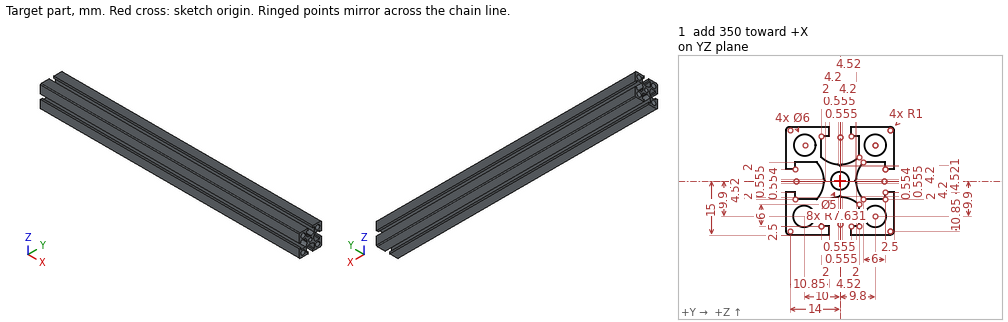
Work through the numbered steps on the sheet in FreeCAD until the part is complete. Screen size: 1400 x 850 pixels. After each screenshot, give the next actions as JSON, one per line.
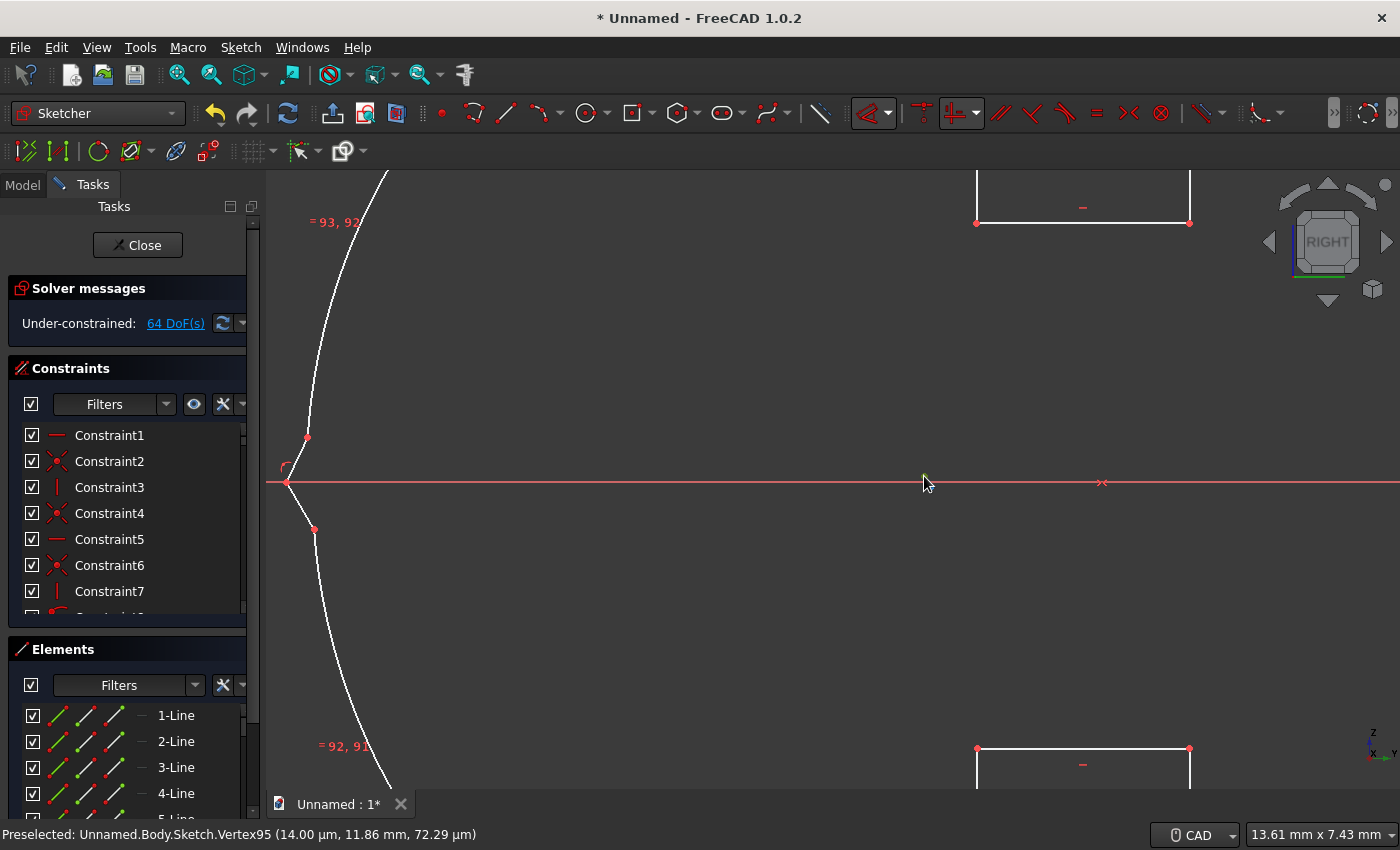
{"action": "scroll", "coordinate": [929, 479], "scroll_direction": "down", "scroll_amount": 9}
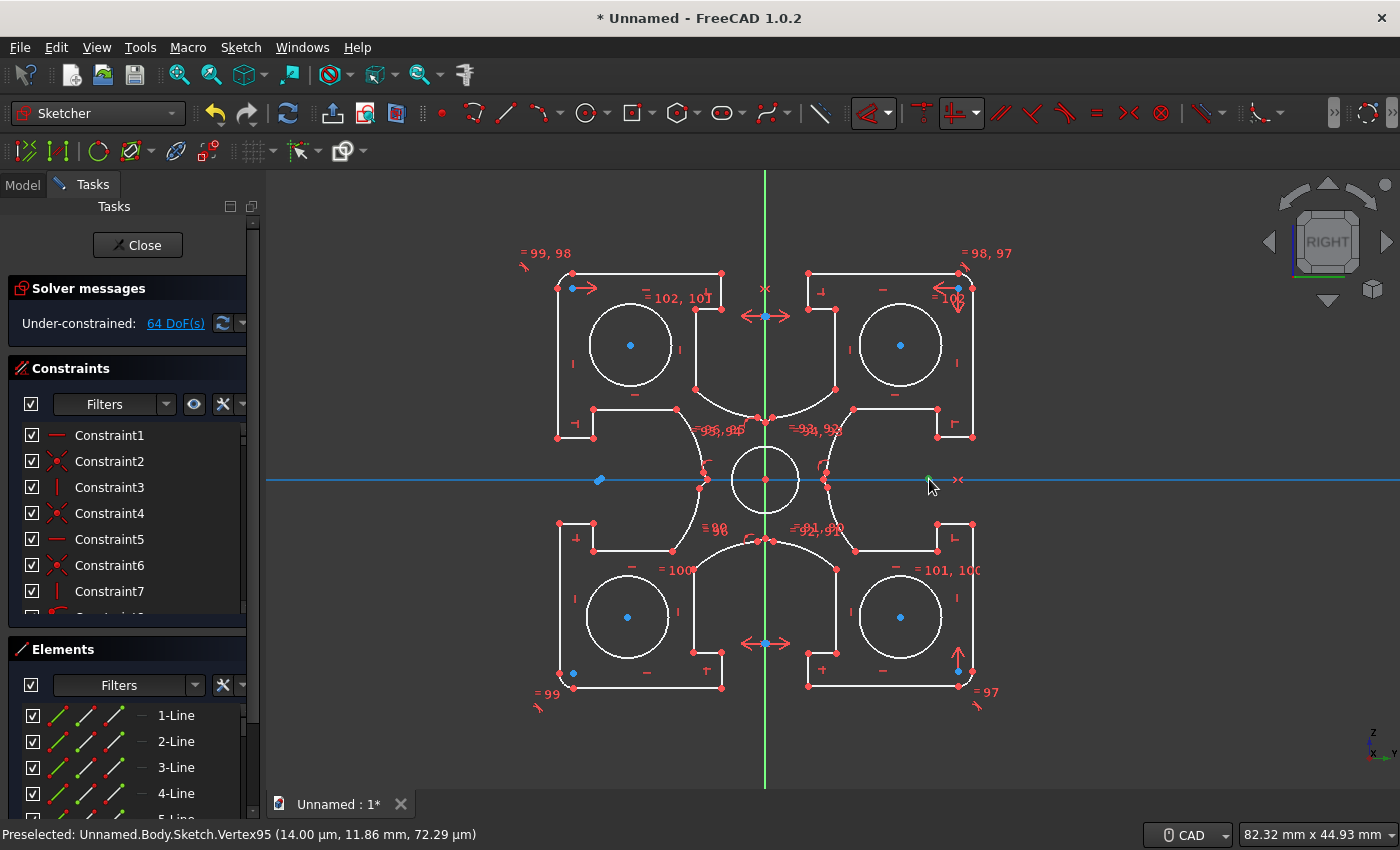
{"action": "scroll", "coordinate": [601, 478], "scroll_direction": "up", "scroll_amount": 6}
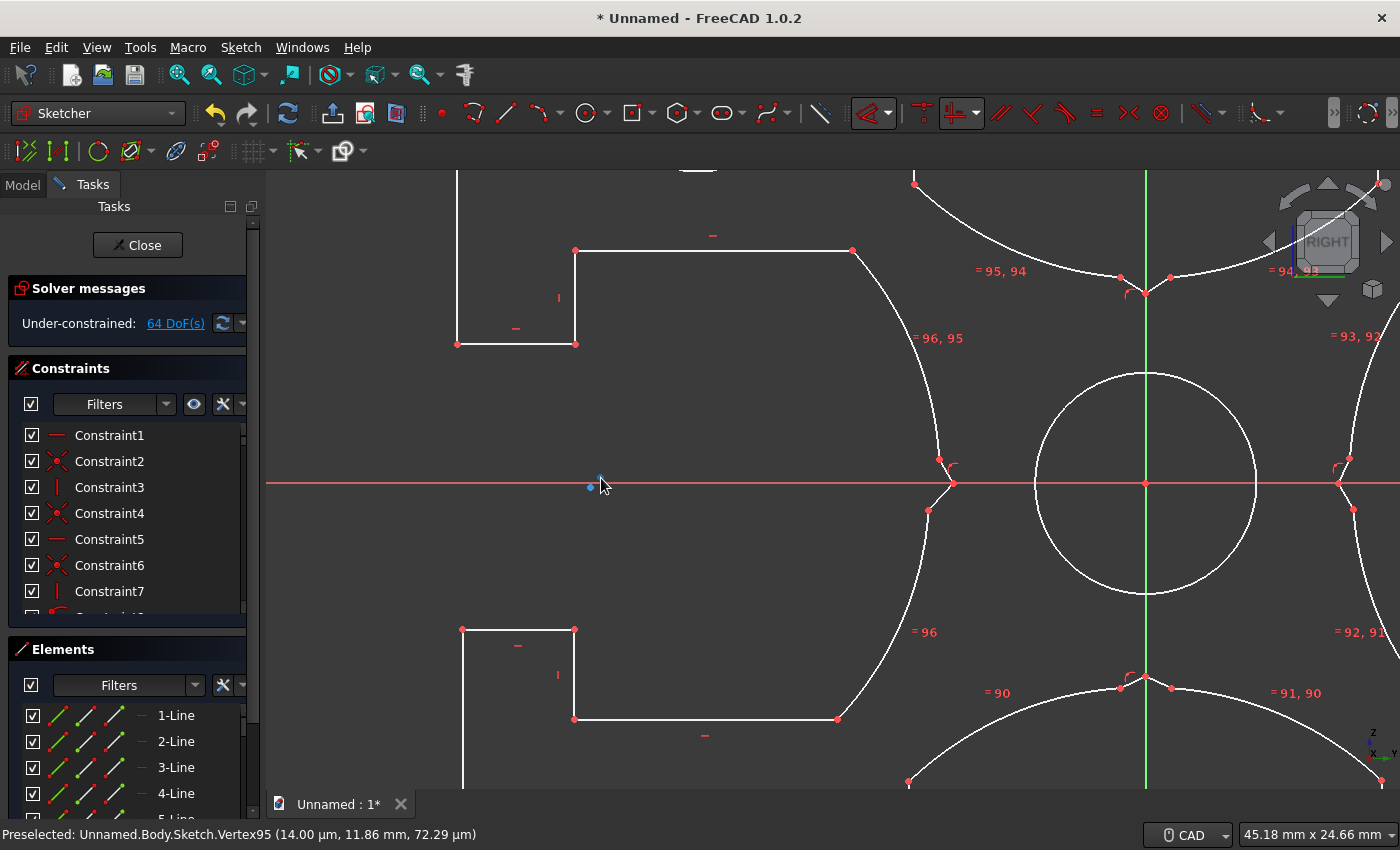
{"action": "left_click", "coordinate": [601, 478]}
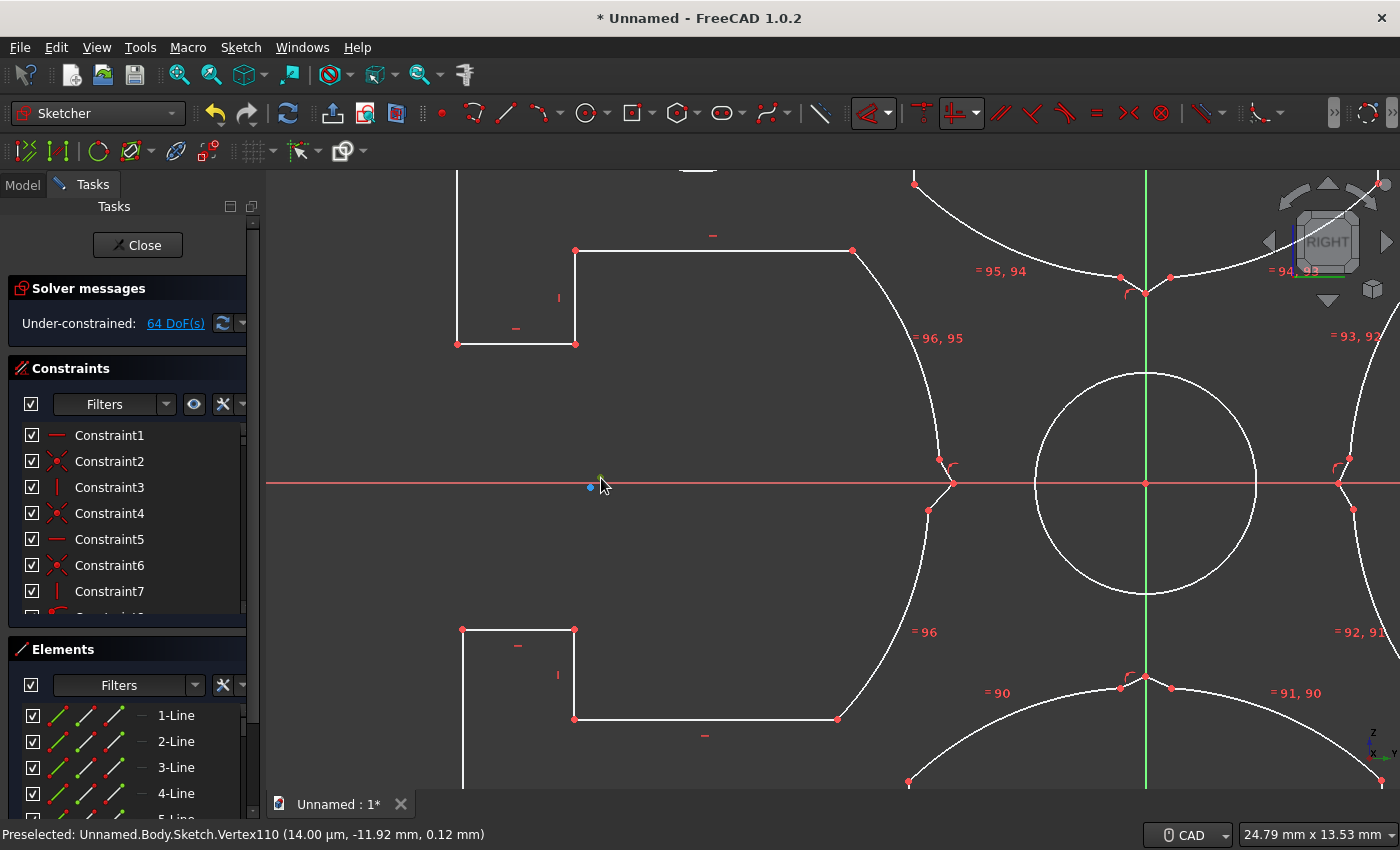
{"action": "left_click", "coordinate": [1146, 721]}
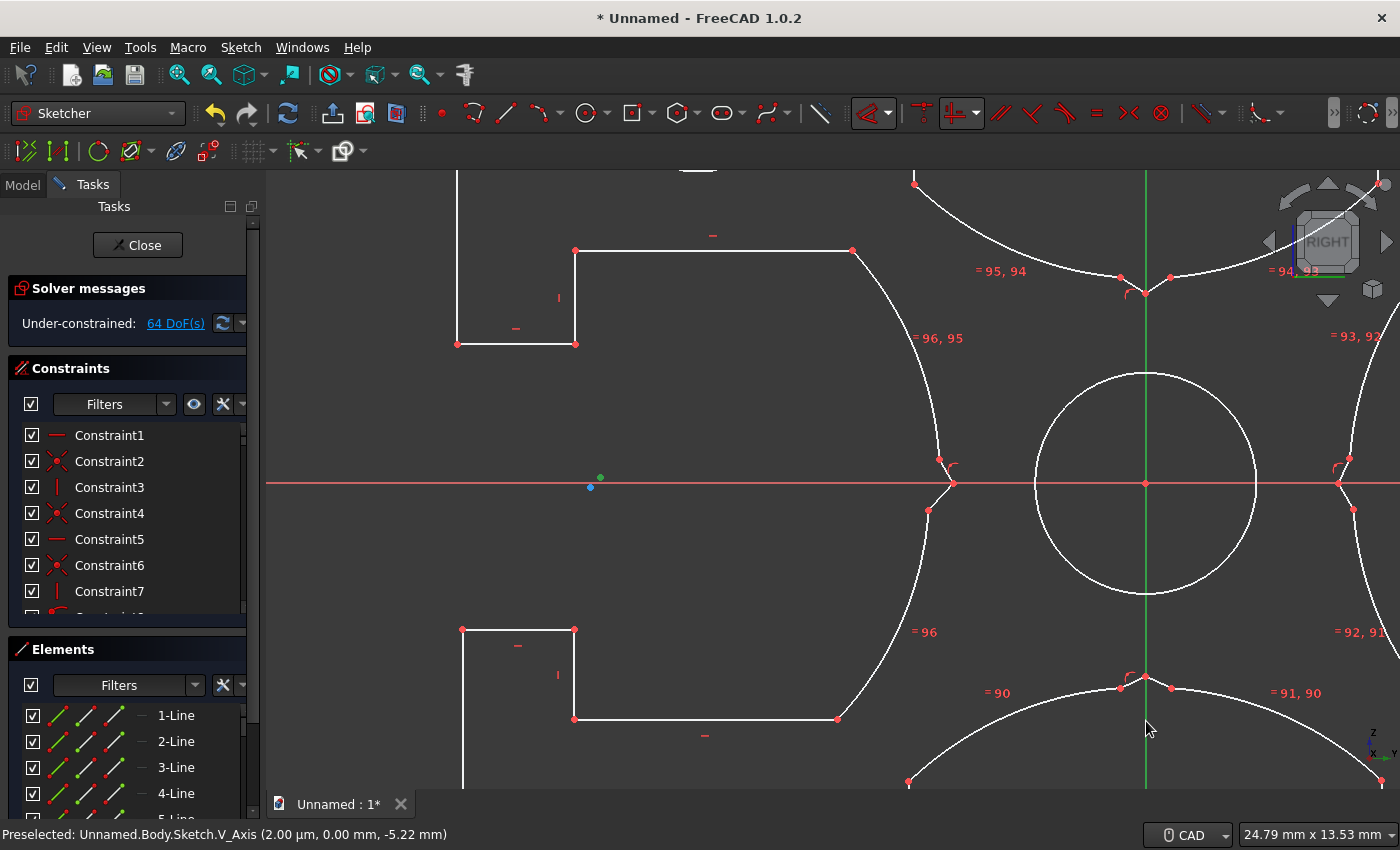
{"action": "left_click", "coordinate": [1130, 114]}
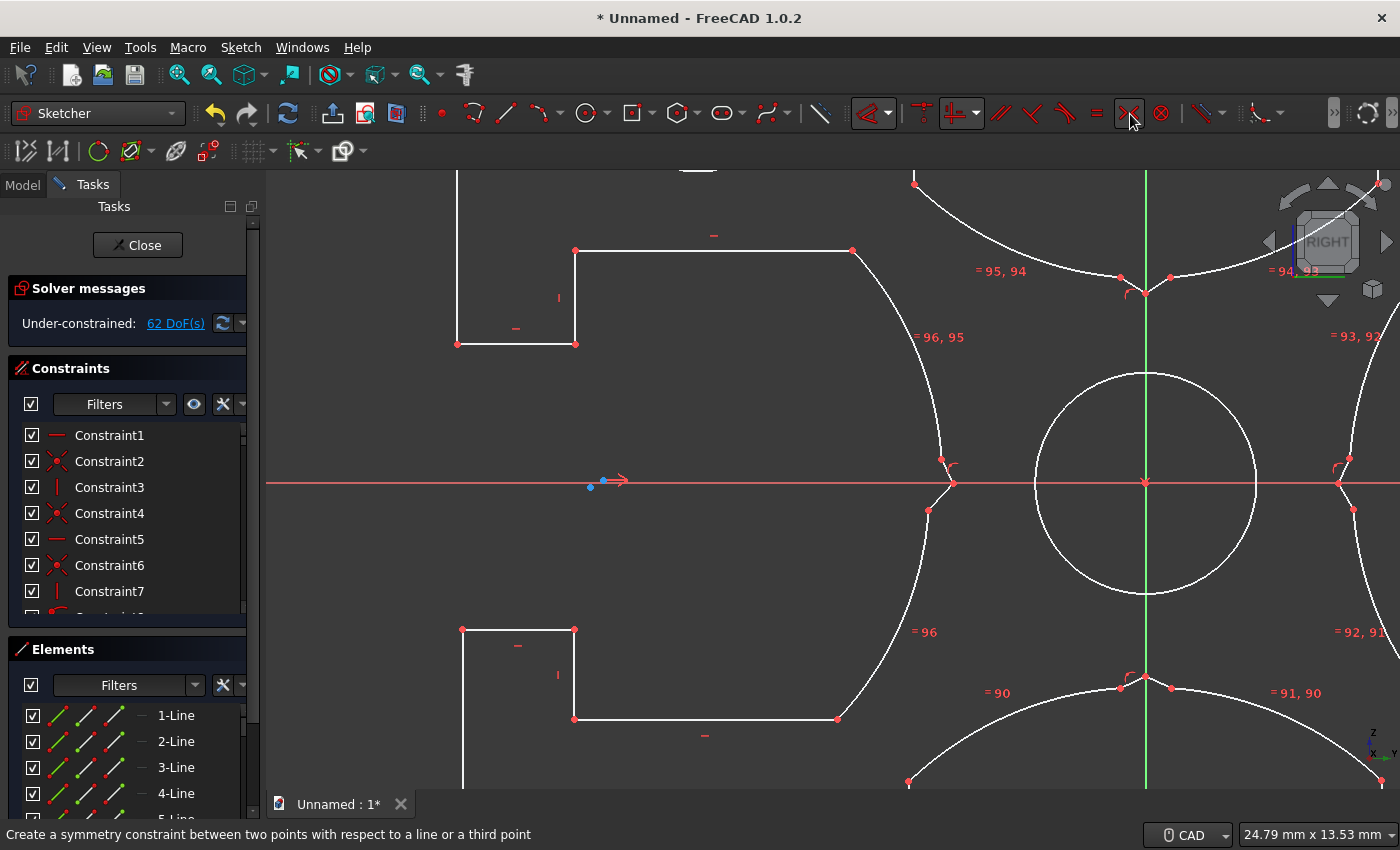
{"action": "scroll", "coordinate": [600, 478], "scroll_direction": "down", "scroll_amount": 6}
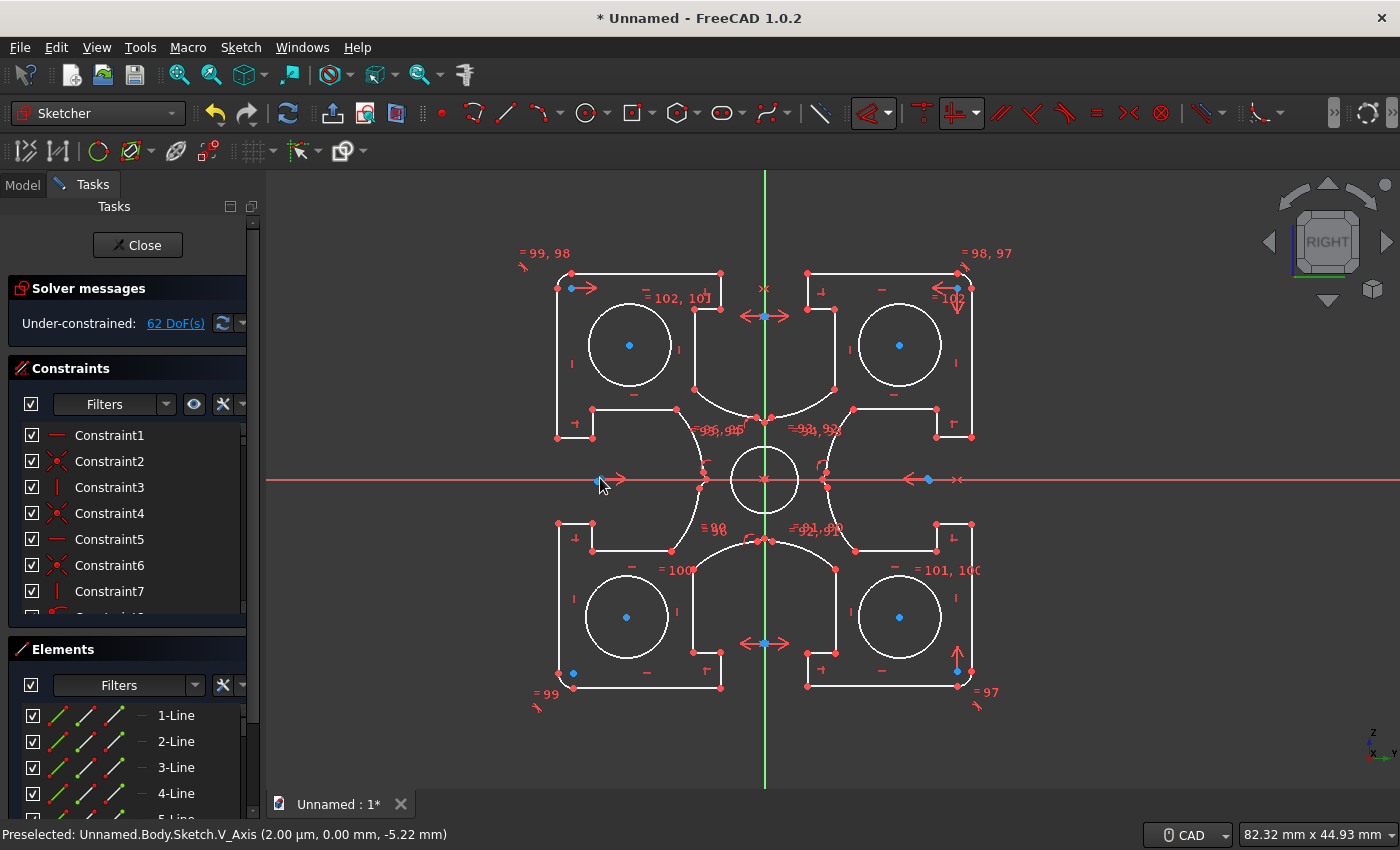
{"action": "scroll", "coordinate": [929, 481], "scroll_direction": "up", "scroll_amount": 9}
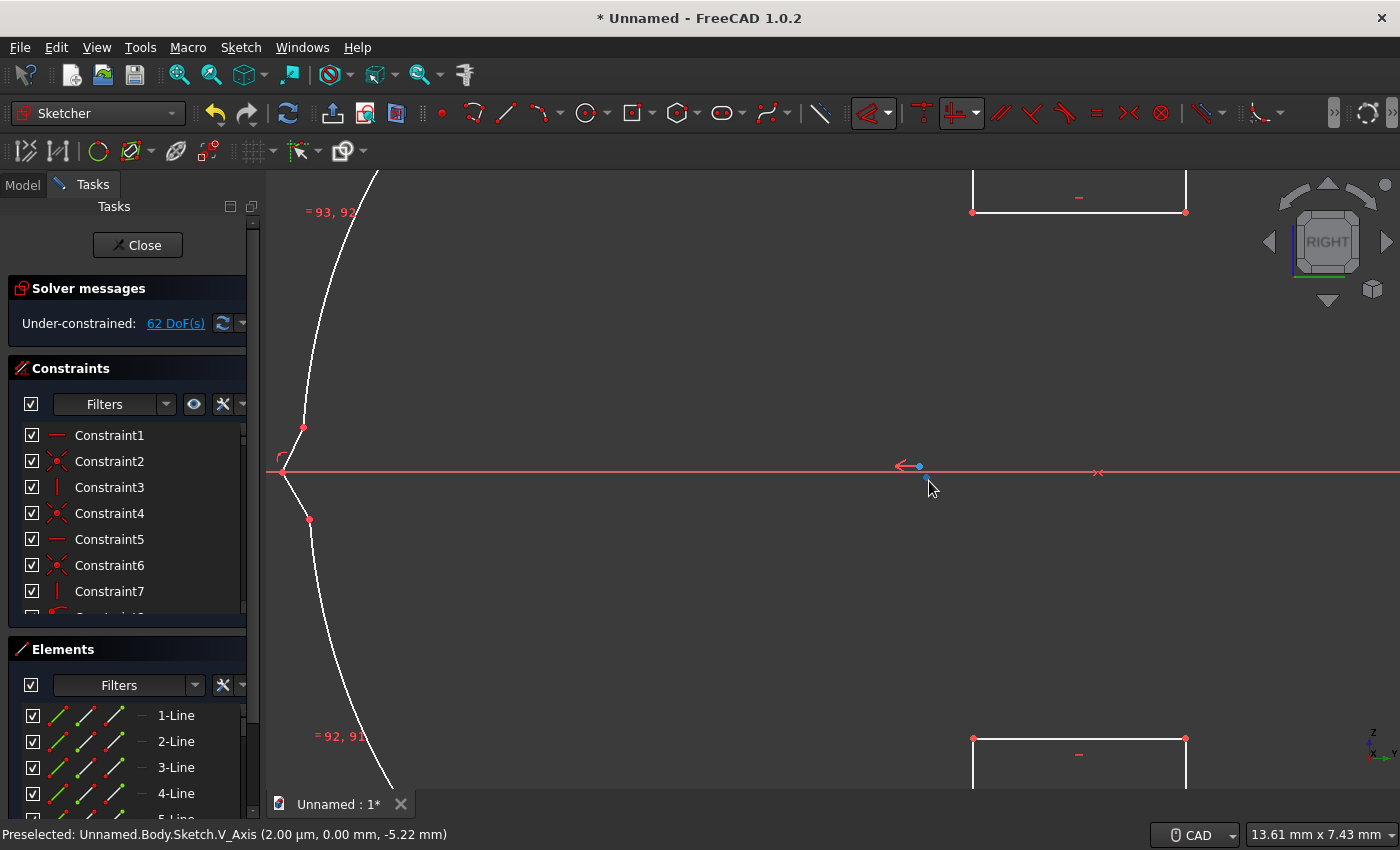
{"action": "left_click", "coordinate": [926, 477]}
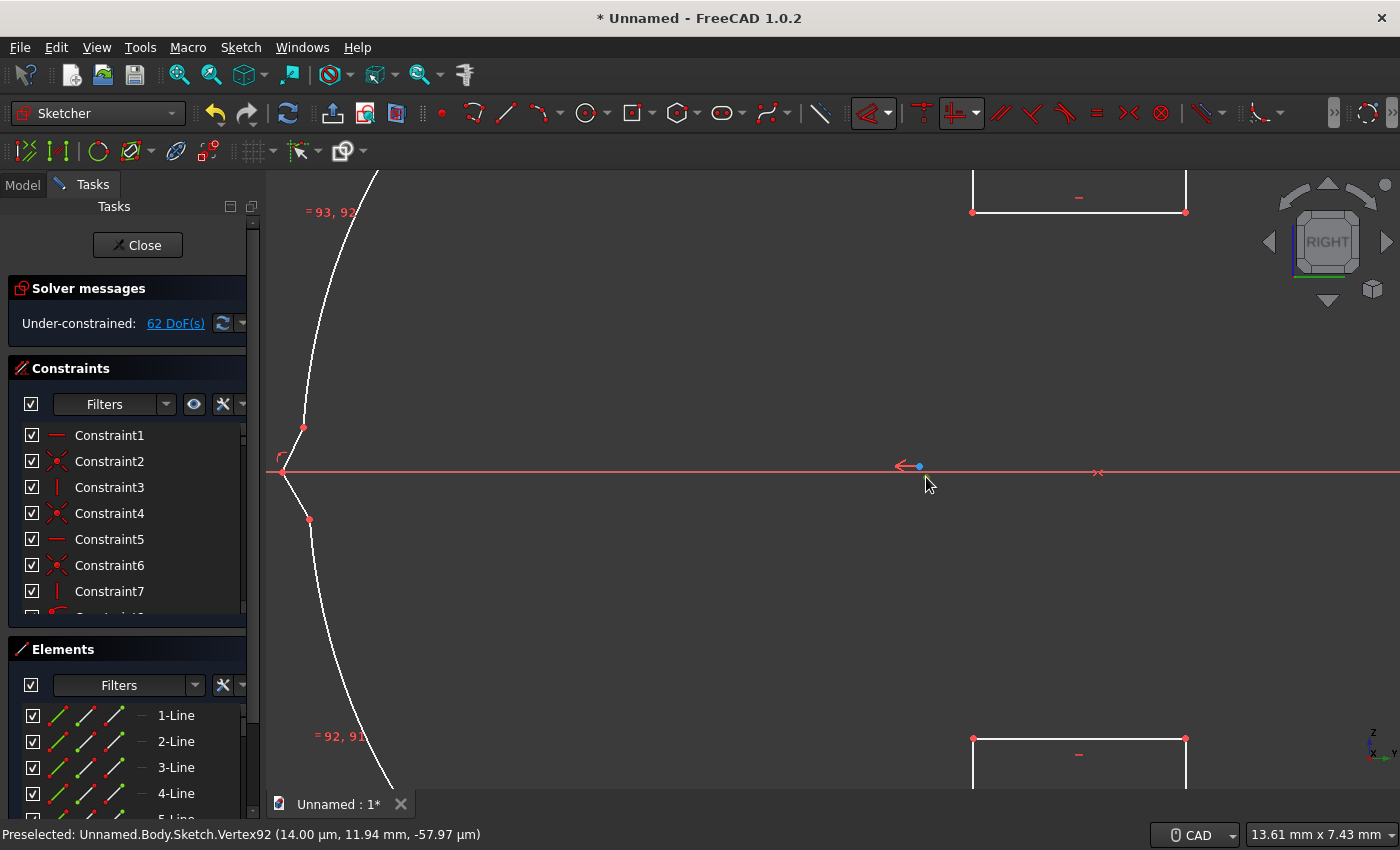
{"action": "scroll", "coordinate": [929, 481], "scroll_direction": "down", "scroll_amount": 9}